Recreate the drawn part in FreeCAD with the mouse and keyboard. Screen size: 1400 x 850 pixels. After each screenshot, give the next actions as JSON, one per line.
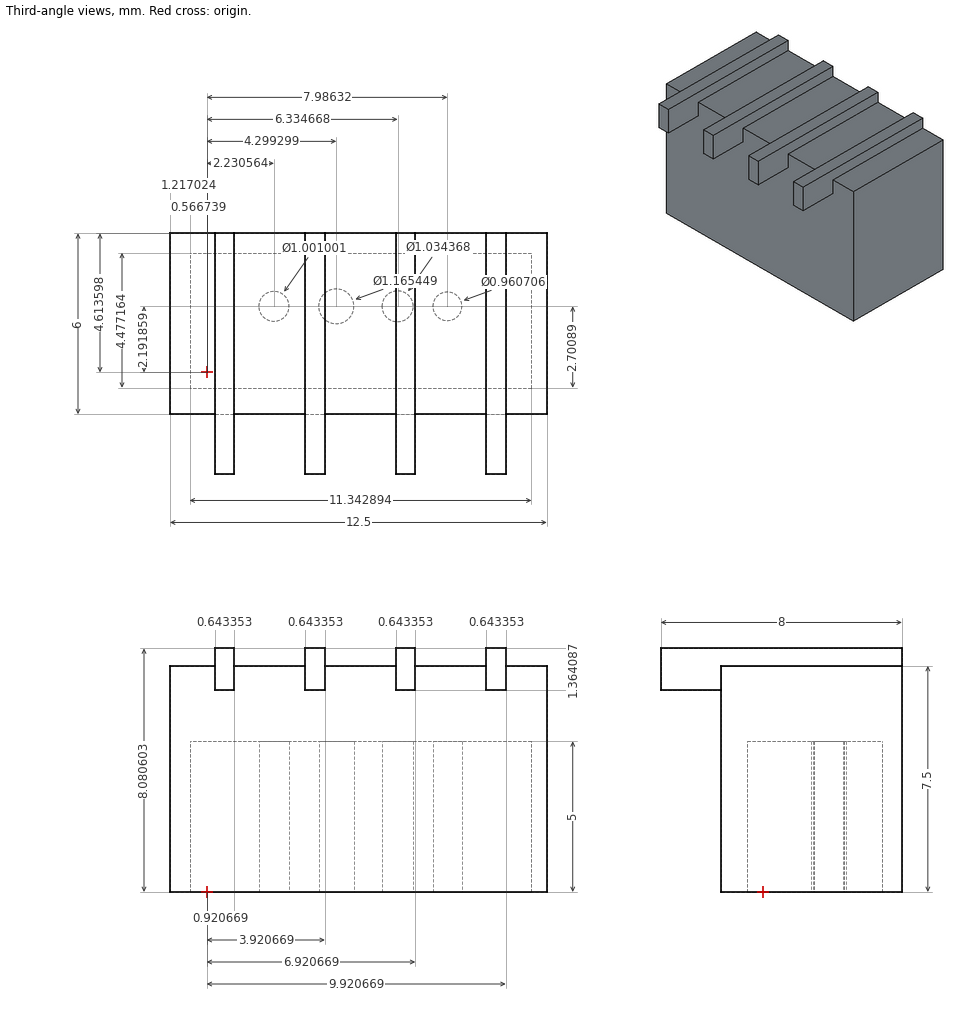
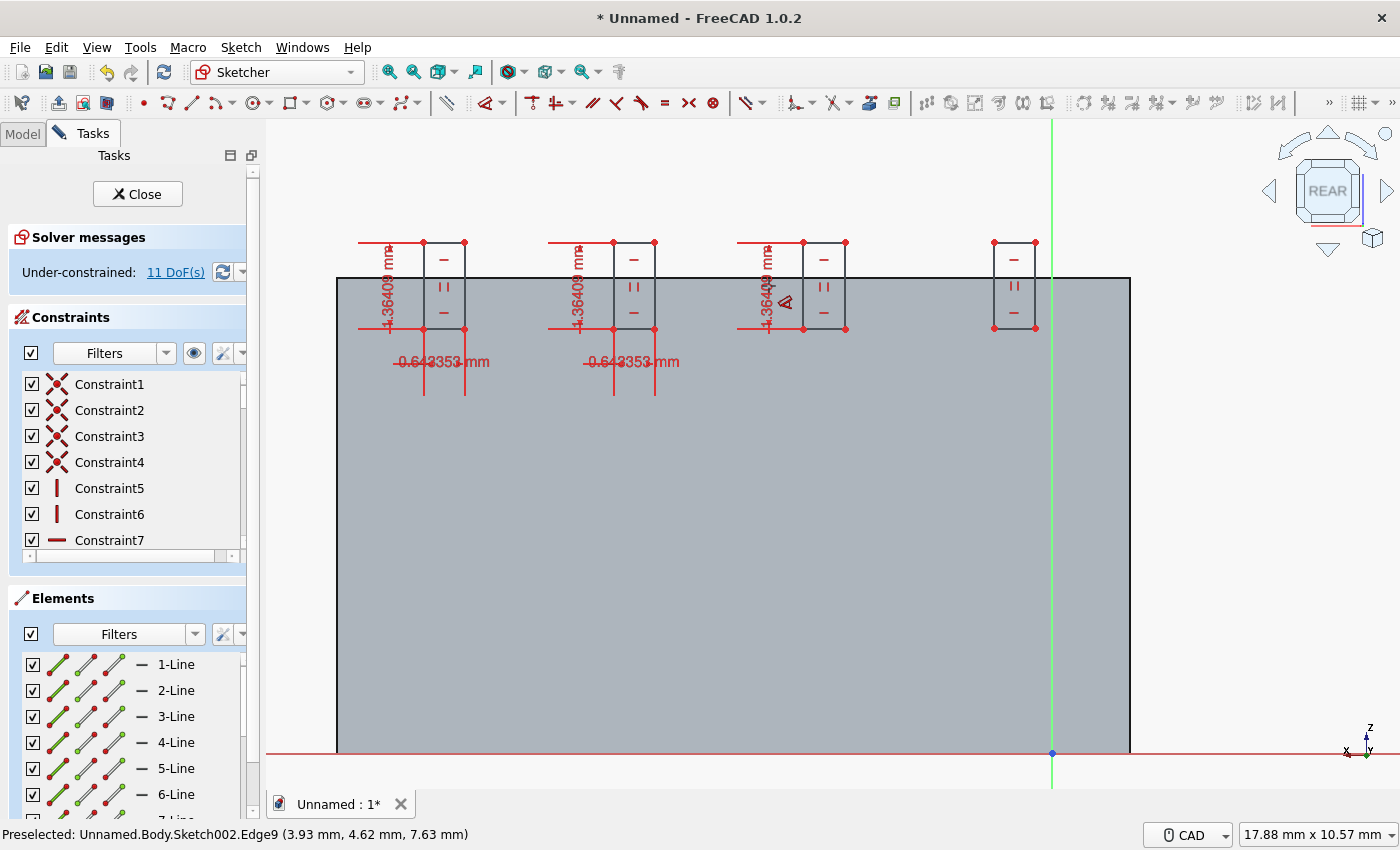
{"action": "left_click", "coordinate": [816, 329]}
{"action": "left_click", "coordinate": [824, 363]}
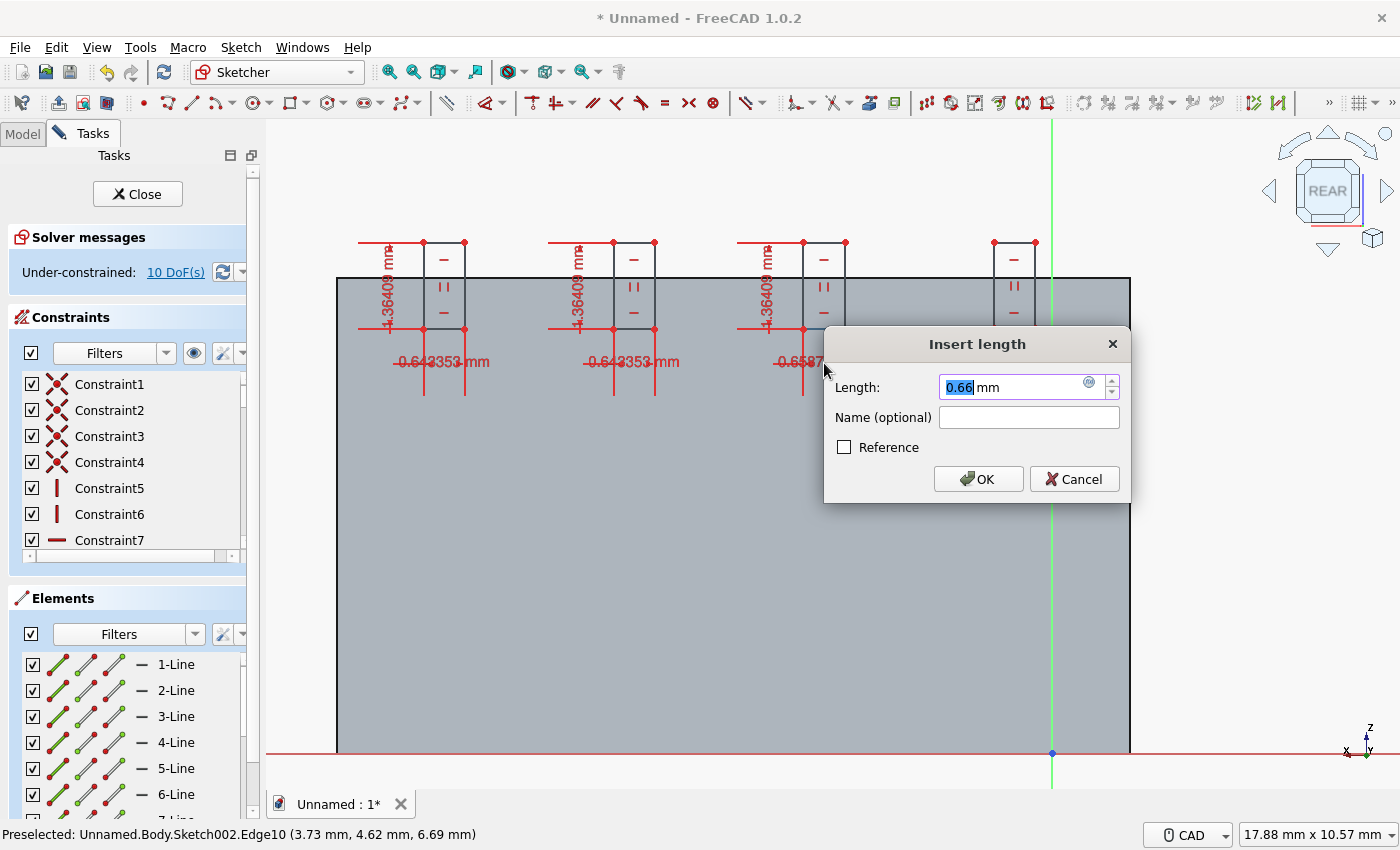
{"action": "type", "text": "0.643353"}
{"action": "key", "text": "Return"}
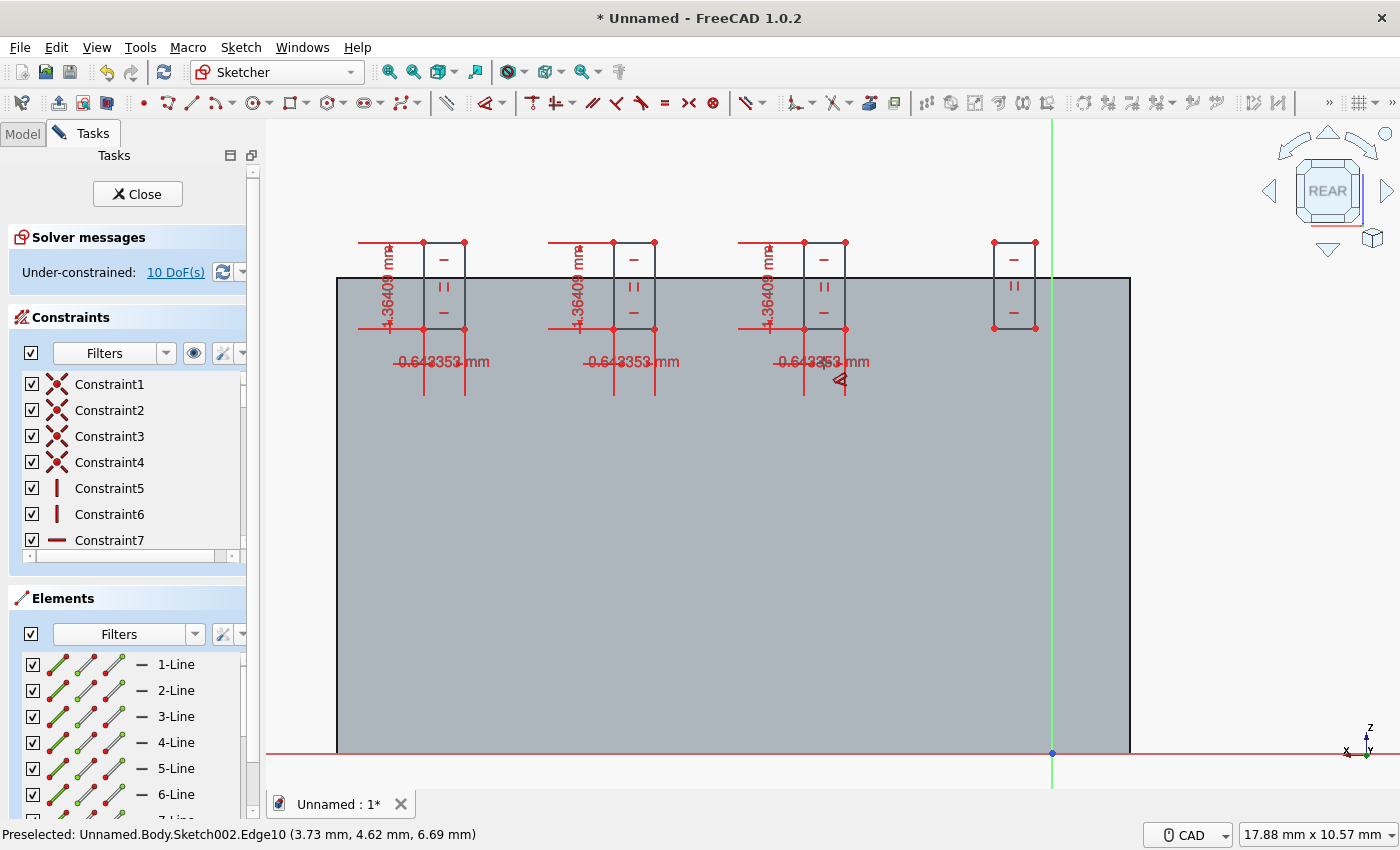
{"action": "left_click", "coordinate": [994, 269]}
{"action": "left_click", "coordinate": [960, 286]}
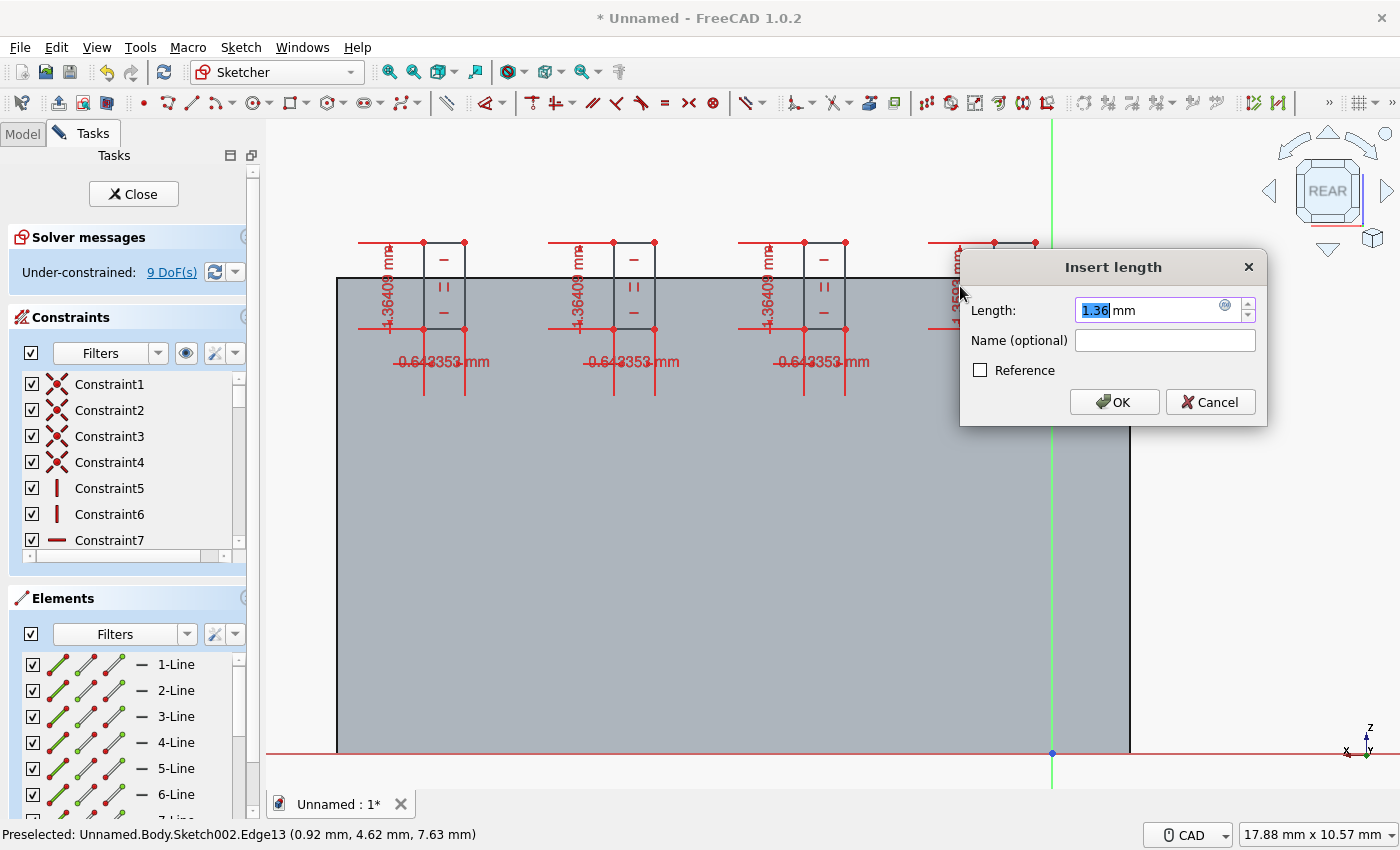
{"action": "type", "text": "1.364087"}
{"action": "key", "text": "Return"}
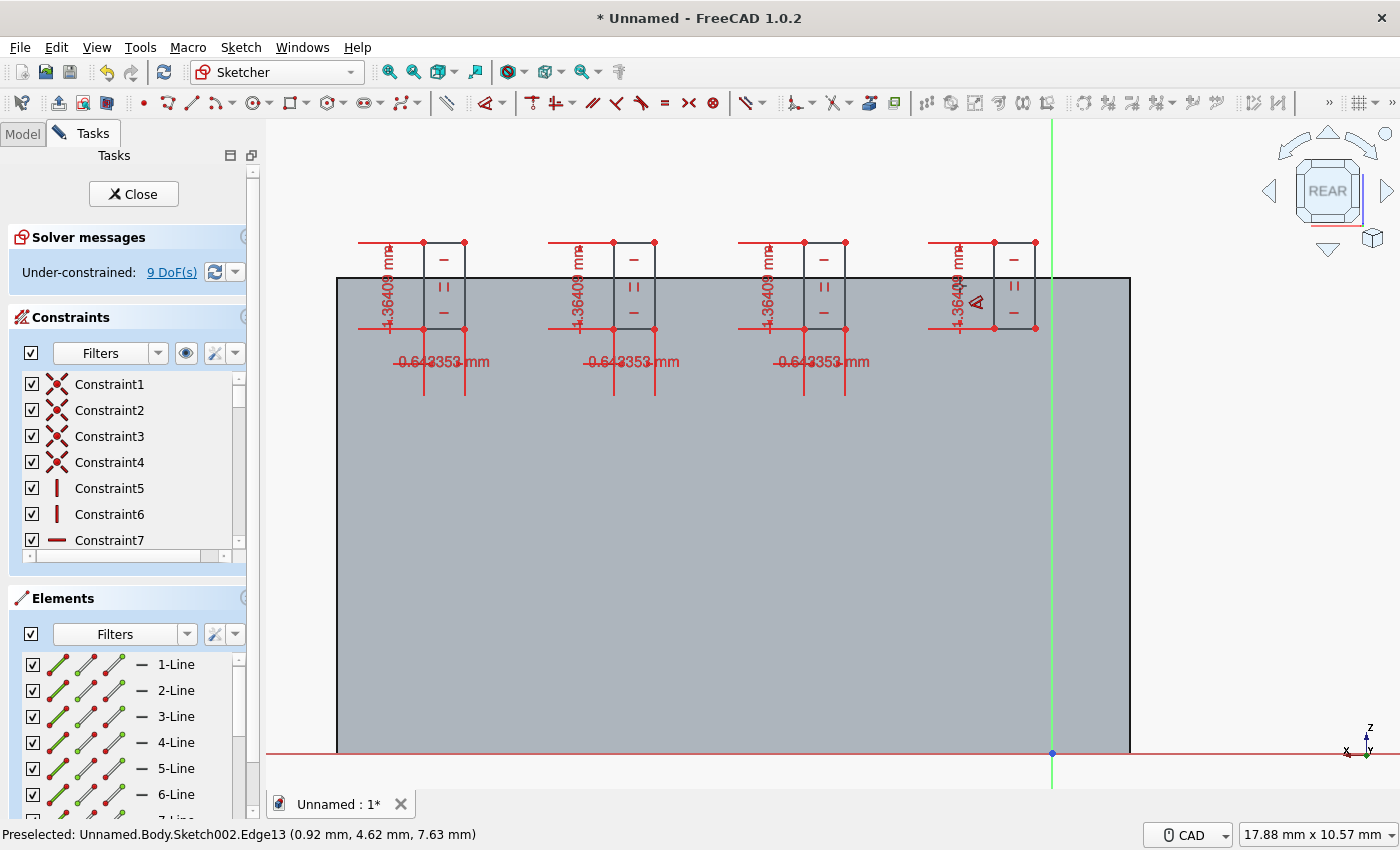
{"action": "left_click", "coordinate": [1007, 329]}
{"action": "left_click", "coordinate": [1015, 363]}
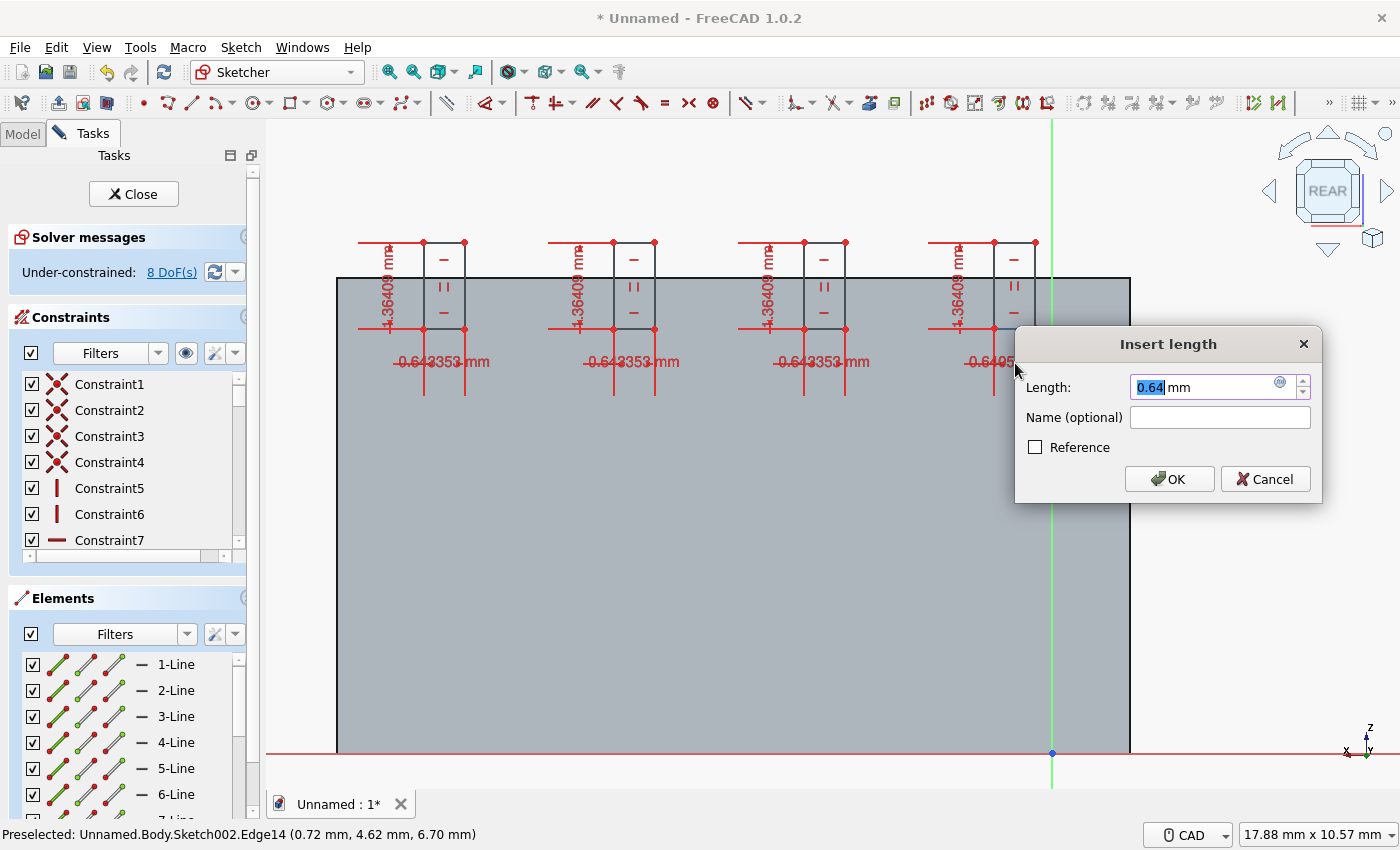
{"action": "type", "text": "0.643353"}
{"action": "key", "text": "Return"}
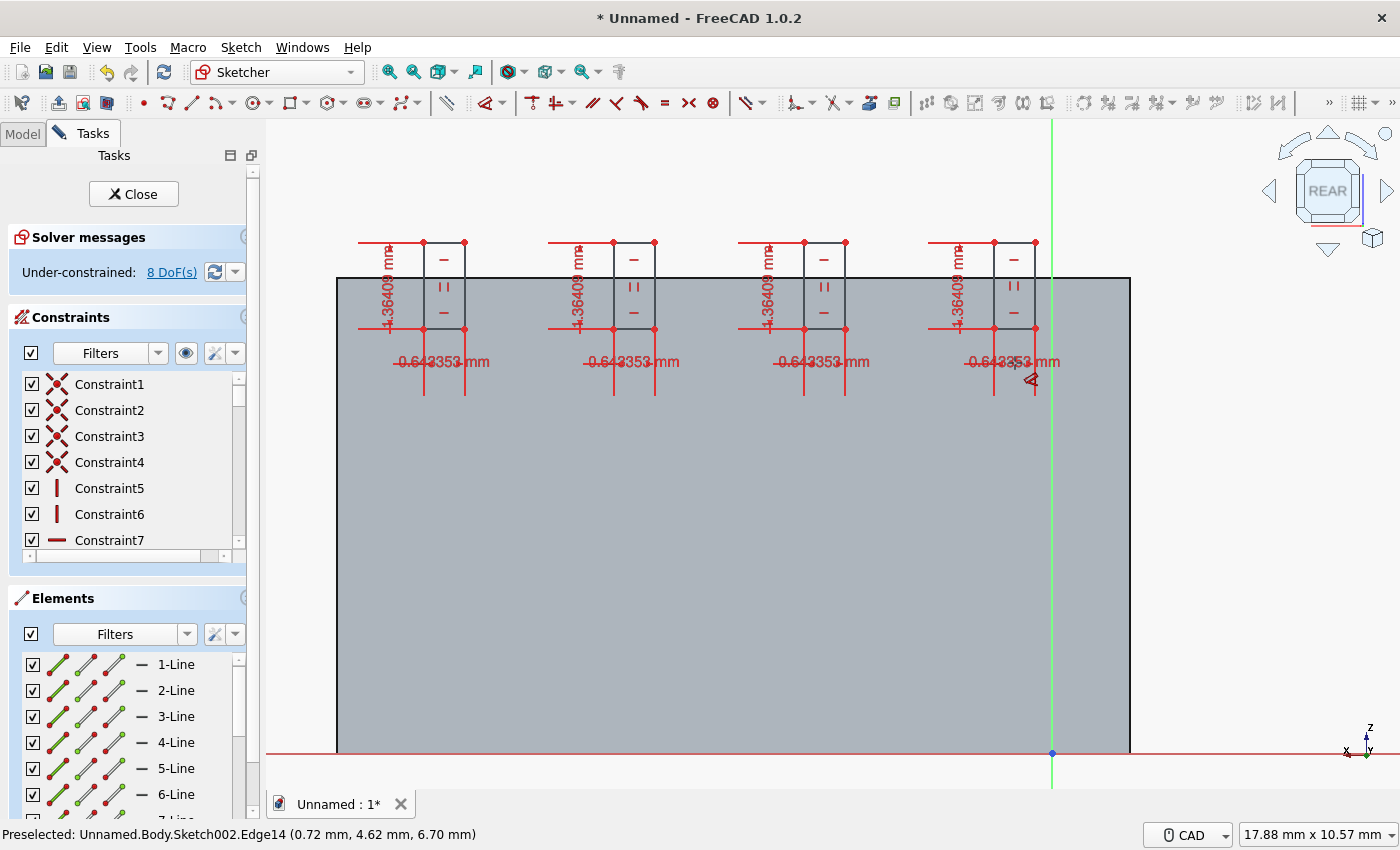
{"action": "left_click", "coordinate": [614, 243]}
{"action": "left_click", "coordinate": [833, 209]}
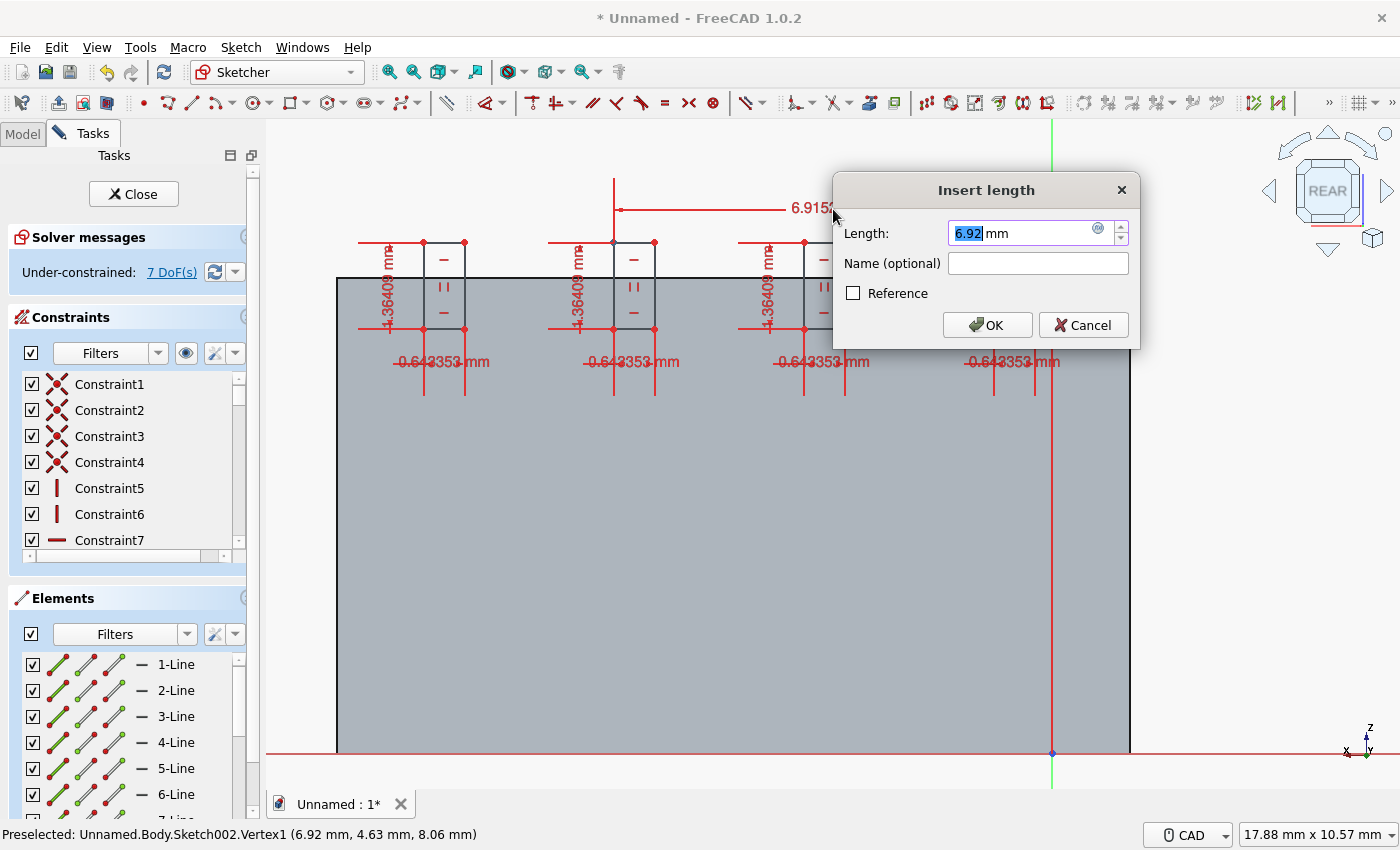
{"action": "type", "text": "6.920669"}
{"action": "key", "text": "Return"}